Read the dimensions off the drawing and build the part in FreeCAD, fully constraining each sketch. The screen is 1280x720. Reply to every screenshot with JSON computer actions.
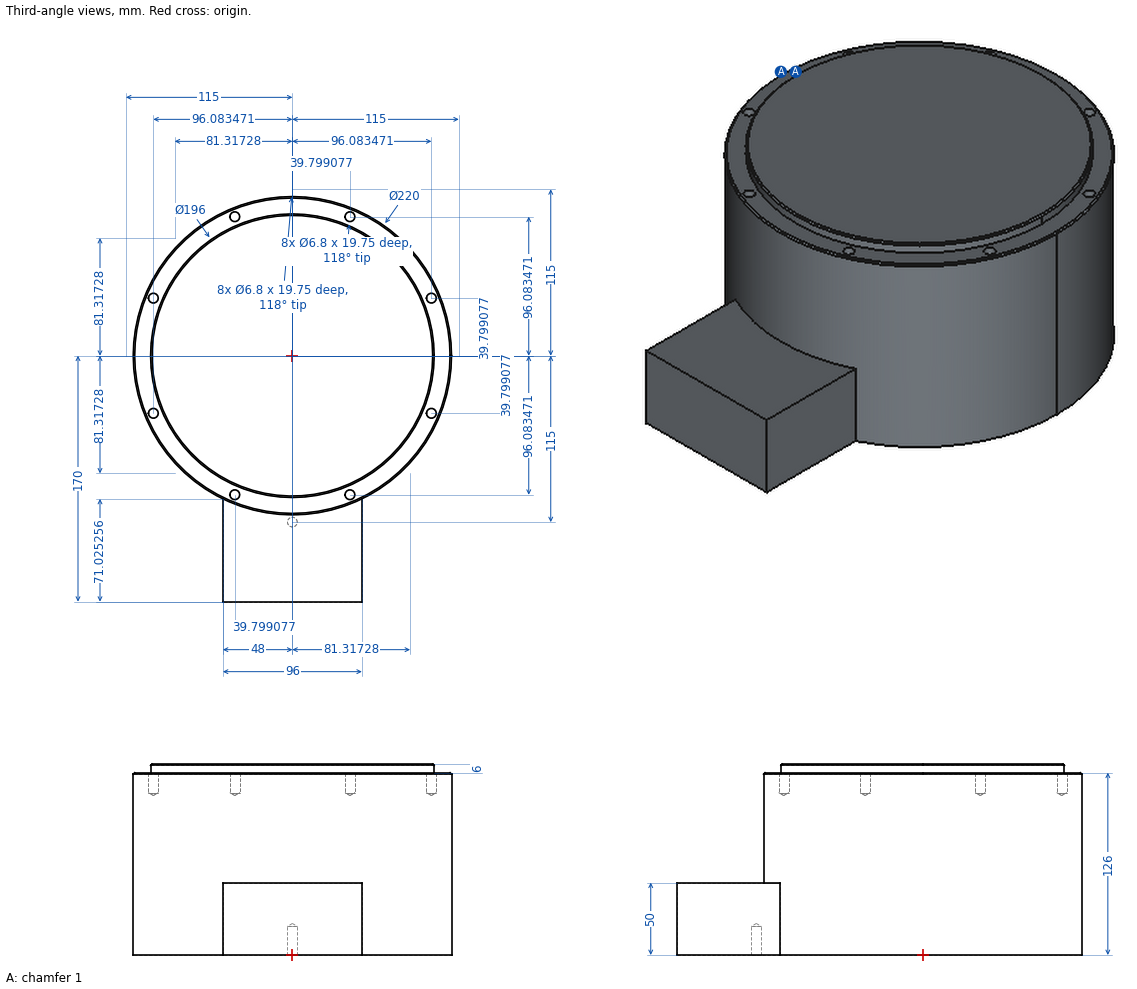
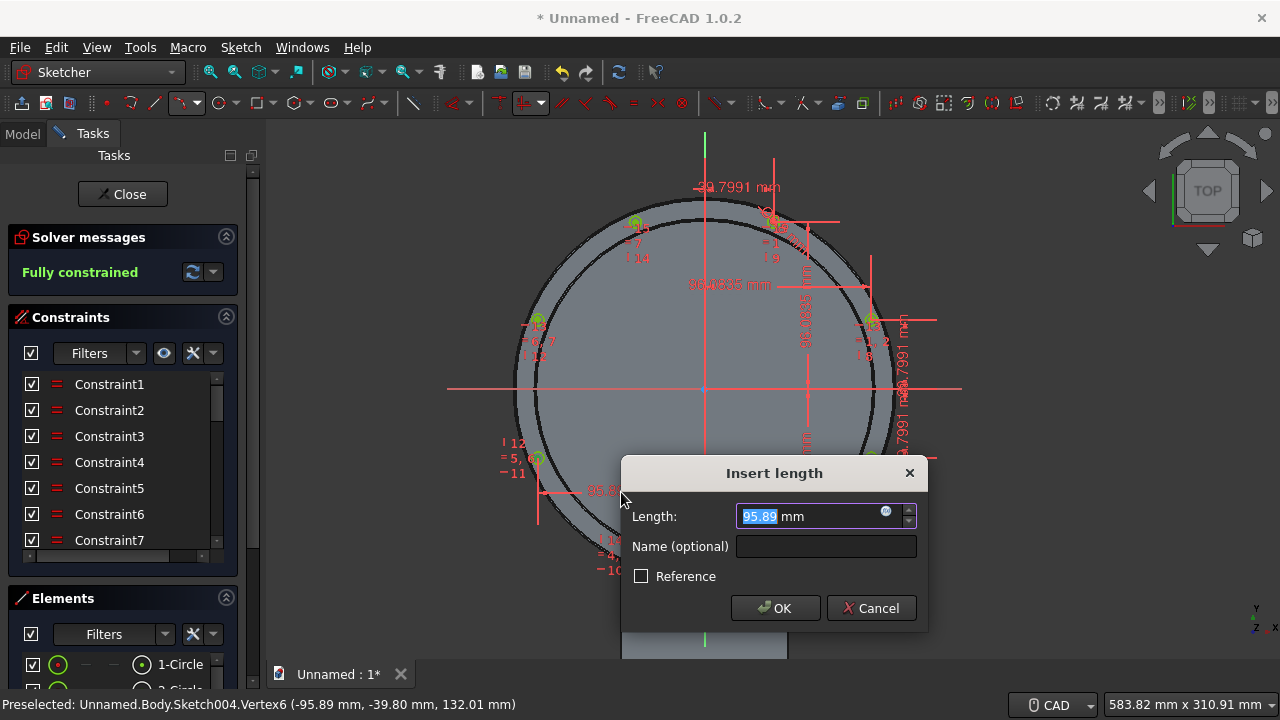
{"action": "type", "text": "96.083471"}
{"action": "key", "text": "Return"}
{"action": "key", "text": "Escape"}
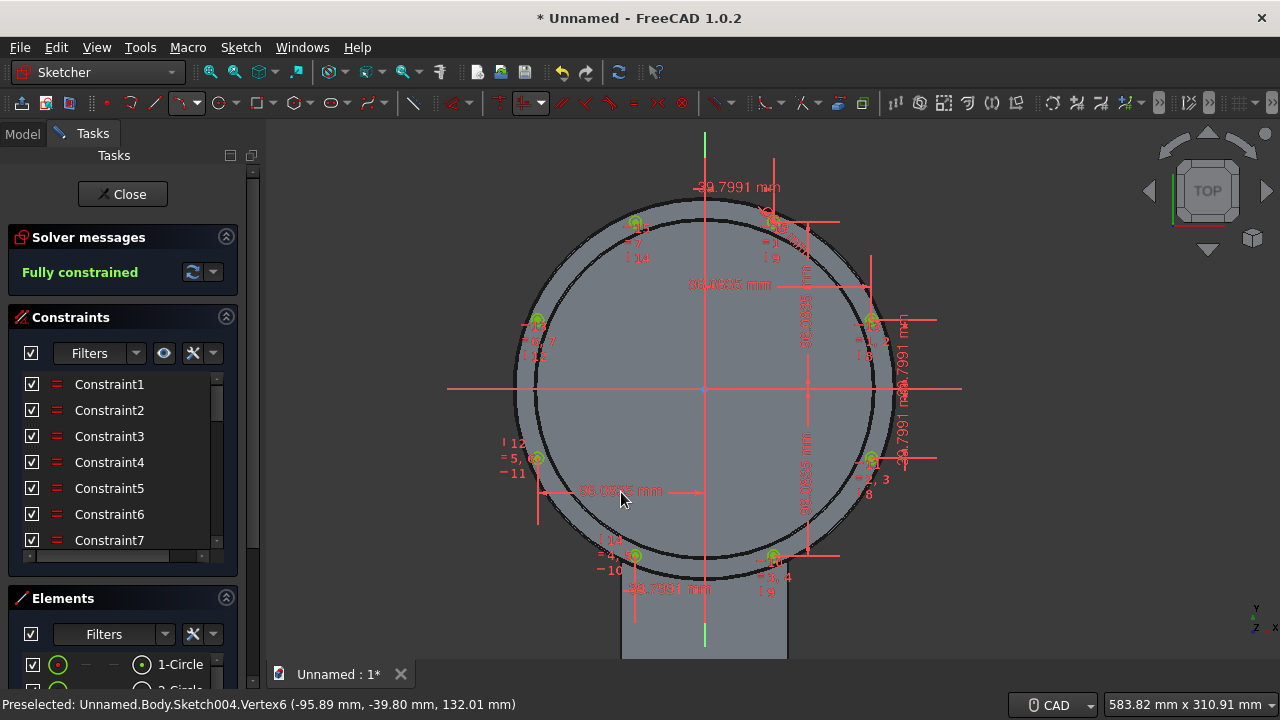
{"action": "left_click", "coordinate": [123, 194]}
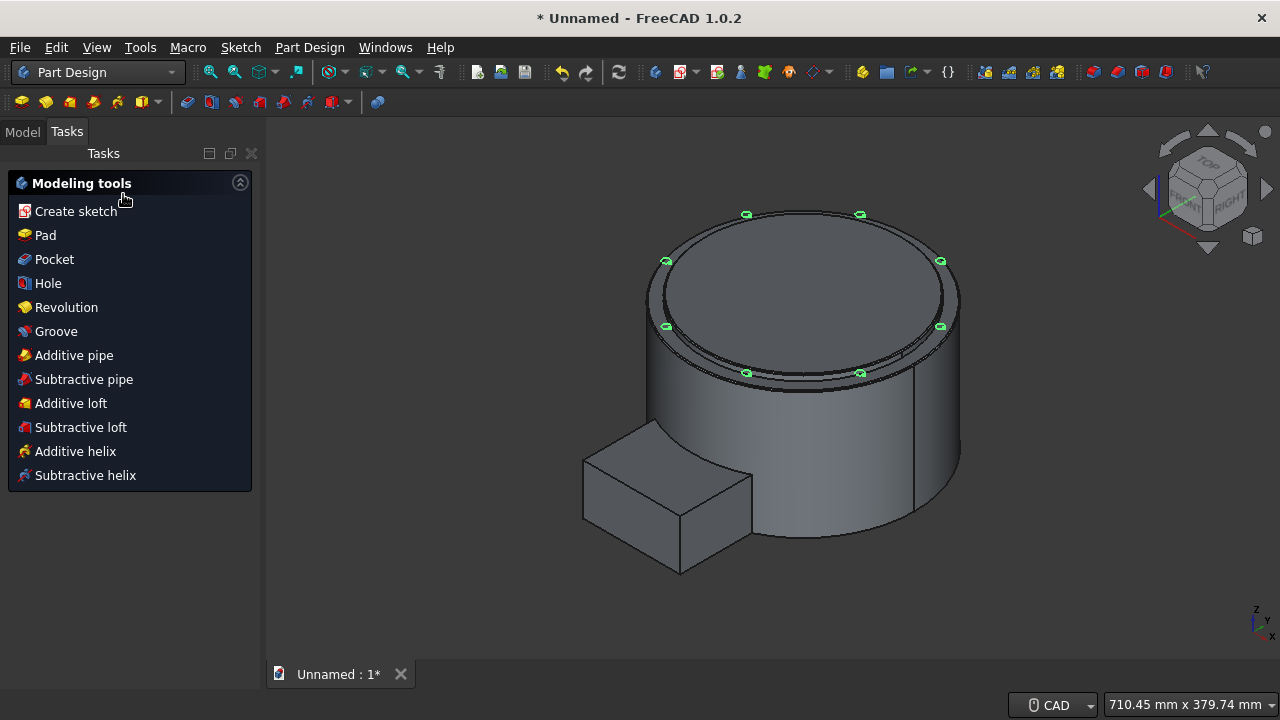
{"action": "left_click", "coordinate": [212, 102]}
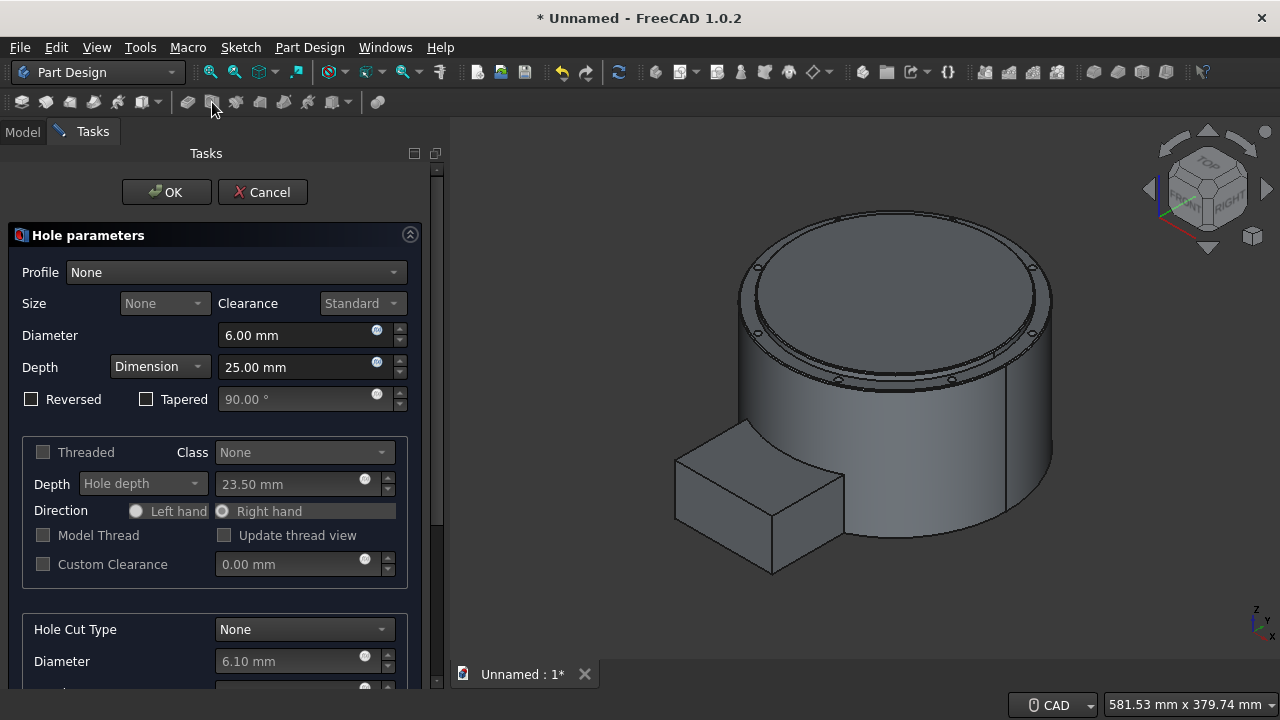
{"action": "triple_click", "coordinate": [305, 335]}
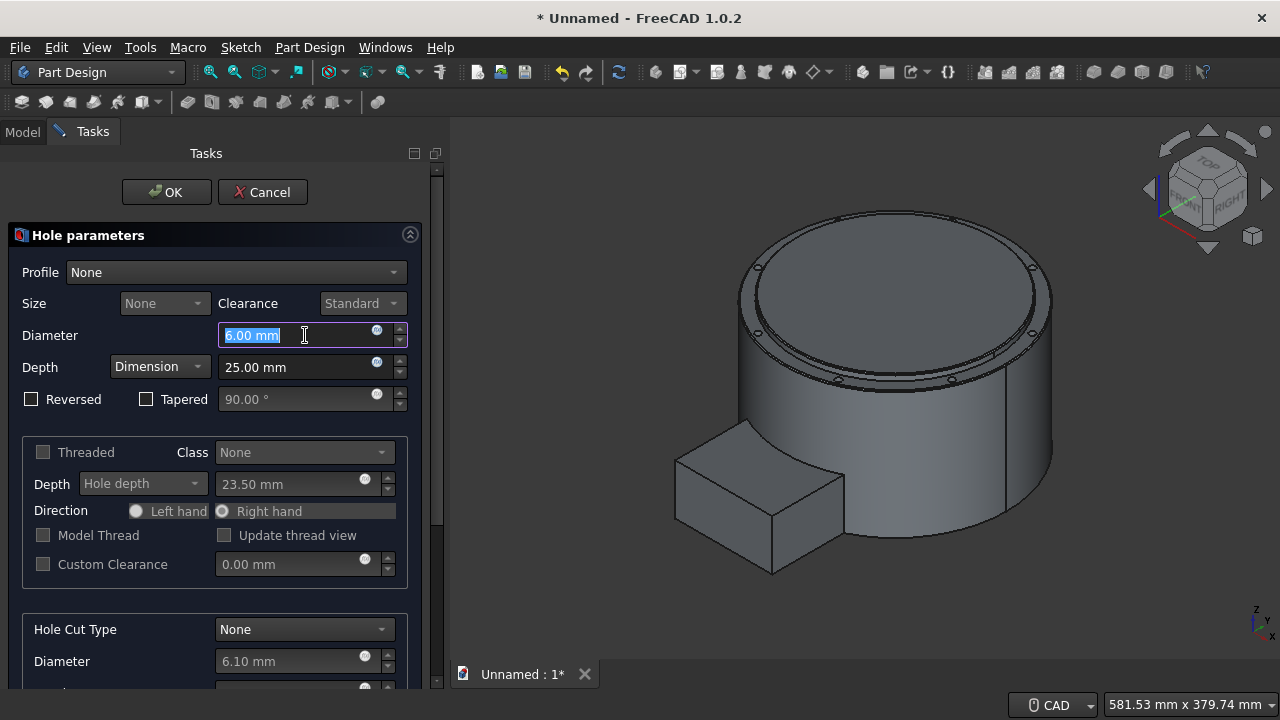
{"action": "type", "text": "6.8"}
{"action": "key", "text": "Tab"}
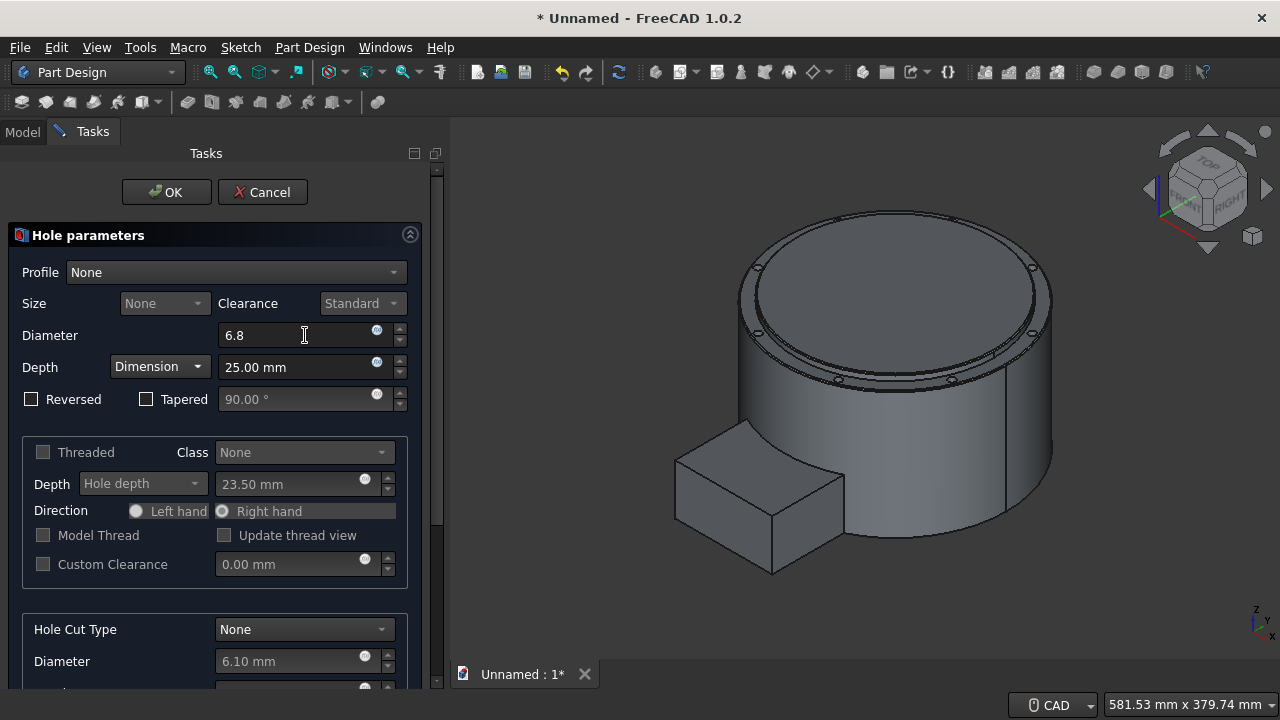
{"action": "triple_click", "coordinate": [305, 367]}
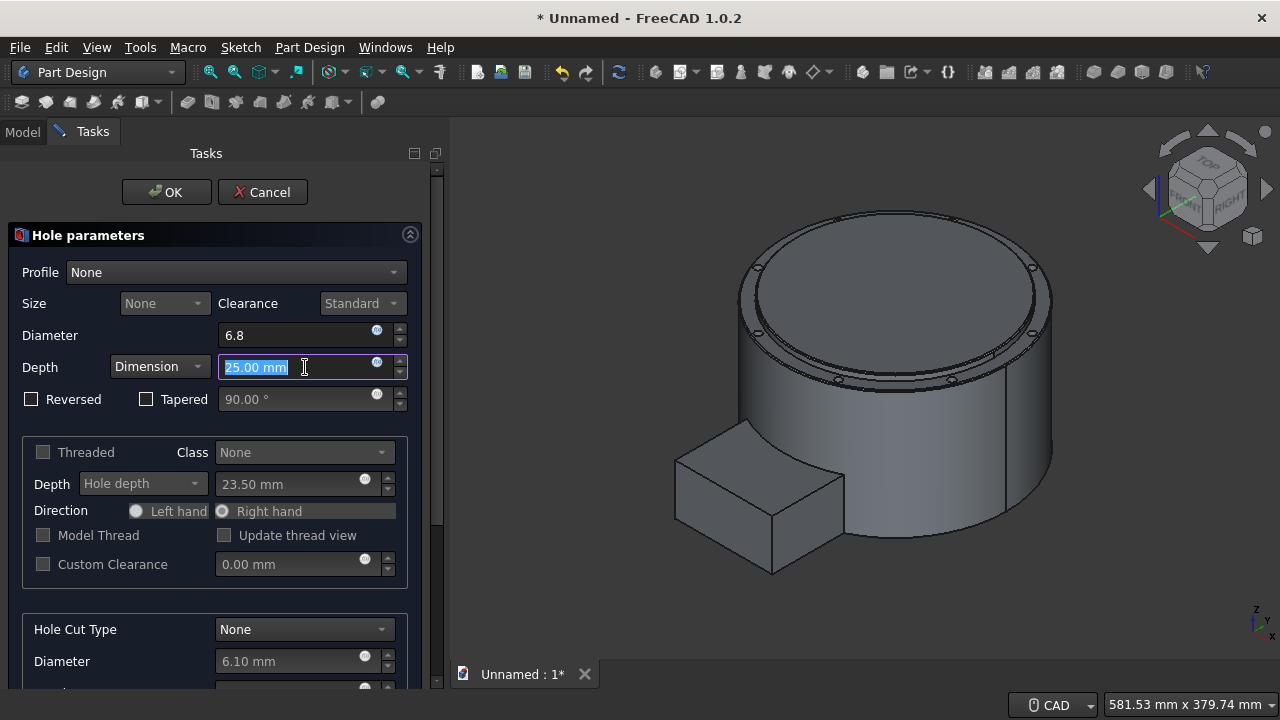
{"action": "type", "text": "19.75"}
{"action": "key", "text": "Tab"}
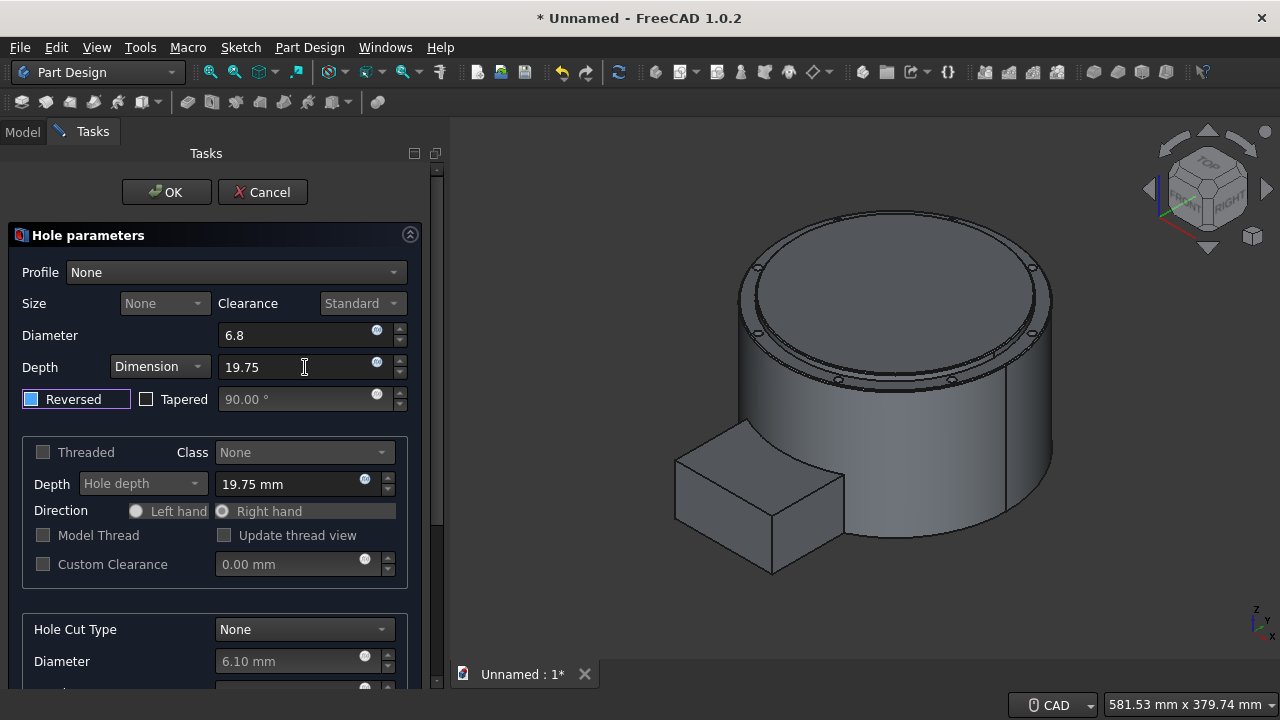
{"action": "left_click", "coordinate": [167, 192]}